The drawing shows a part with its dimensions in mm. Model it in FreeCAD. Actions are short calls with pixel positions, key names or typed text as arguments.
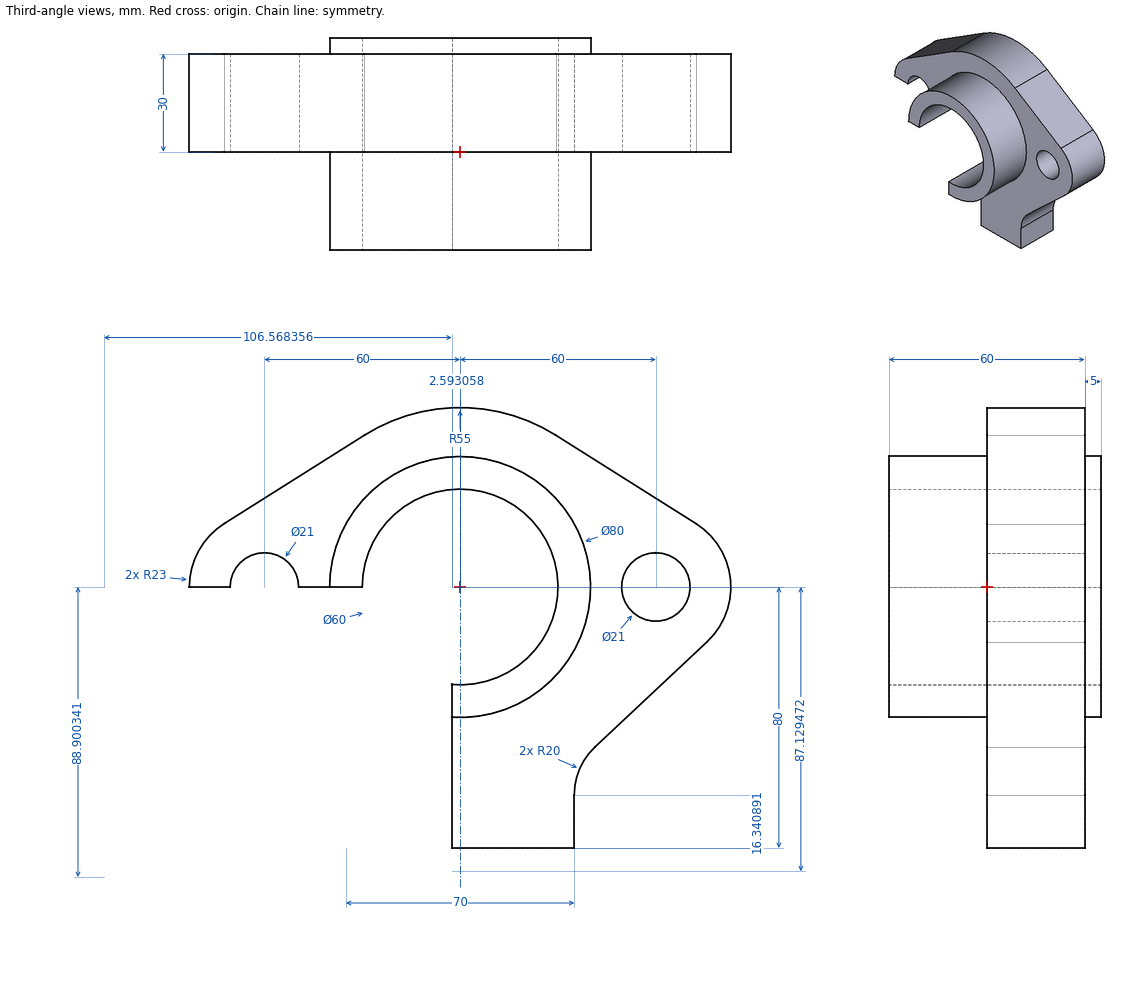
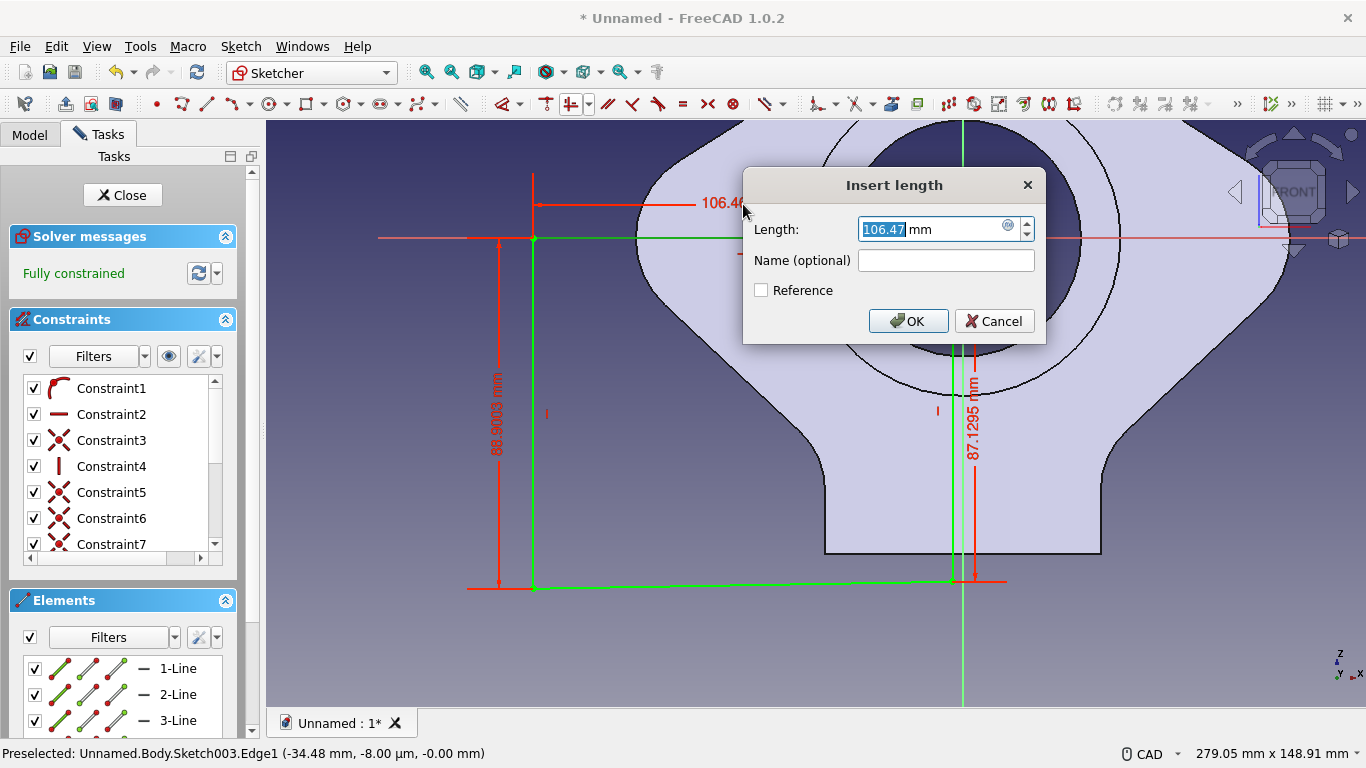
text(106.568356)
key(Return)
key(Escape)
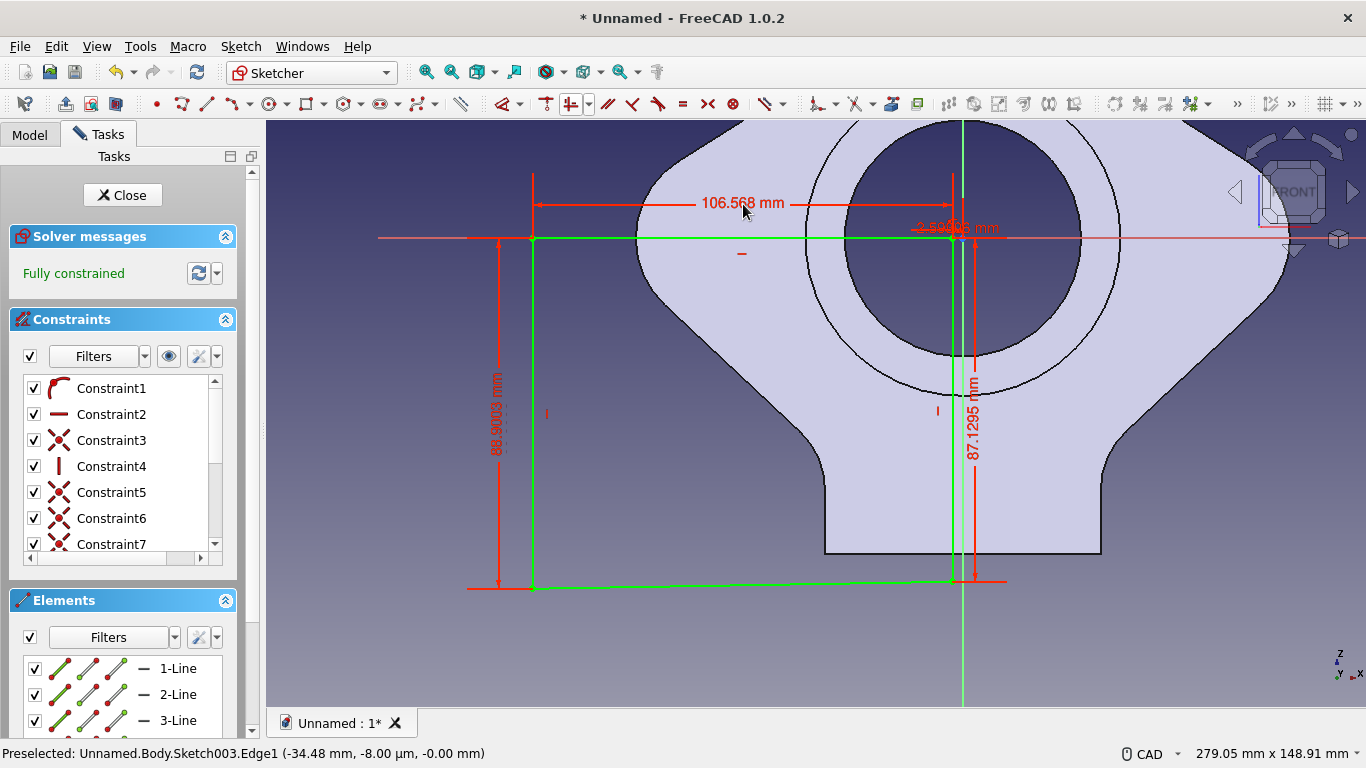
click(123, 195)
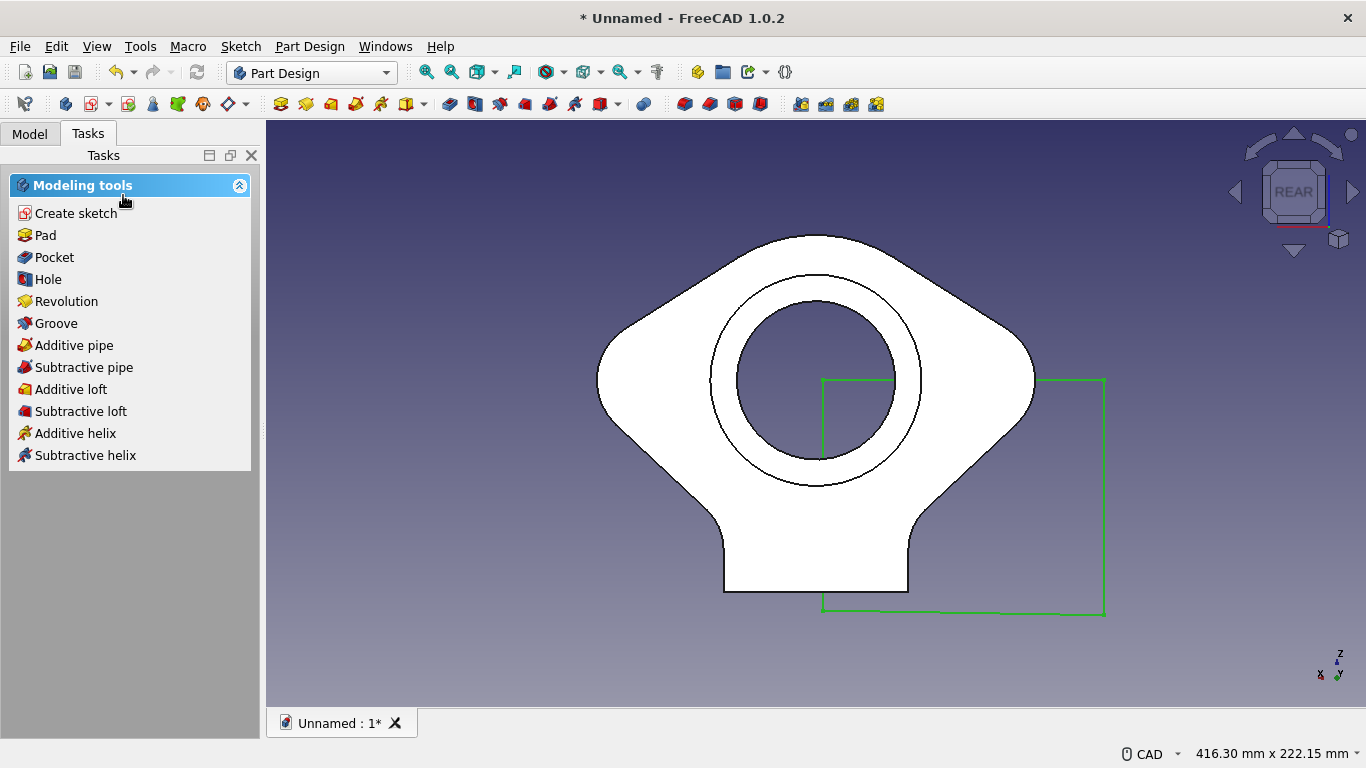
click(450, 104)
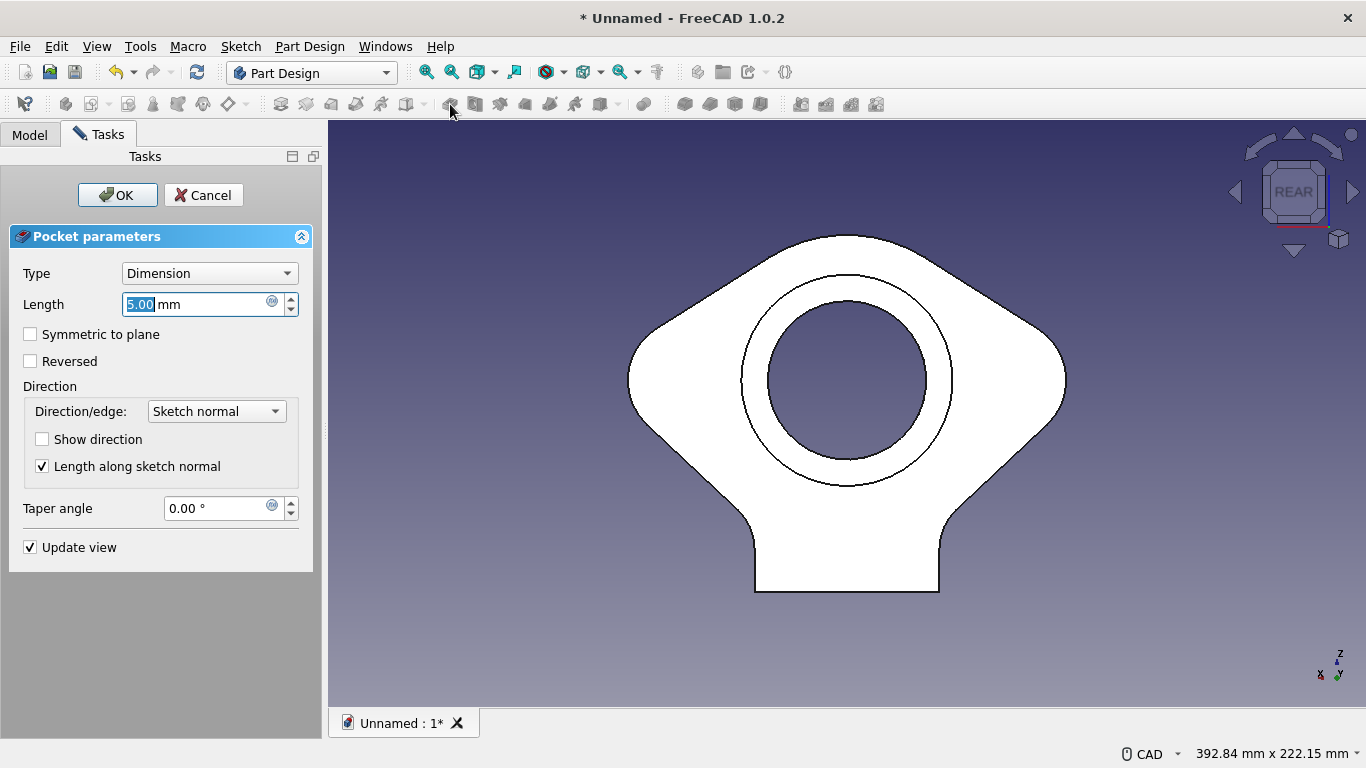
click(210, 274)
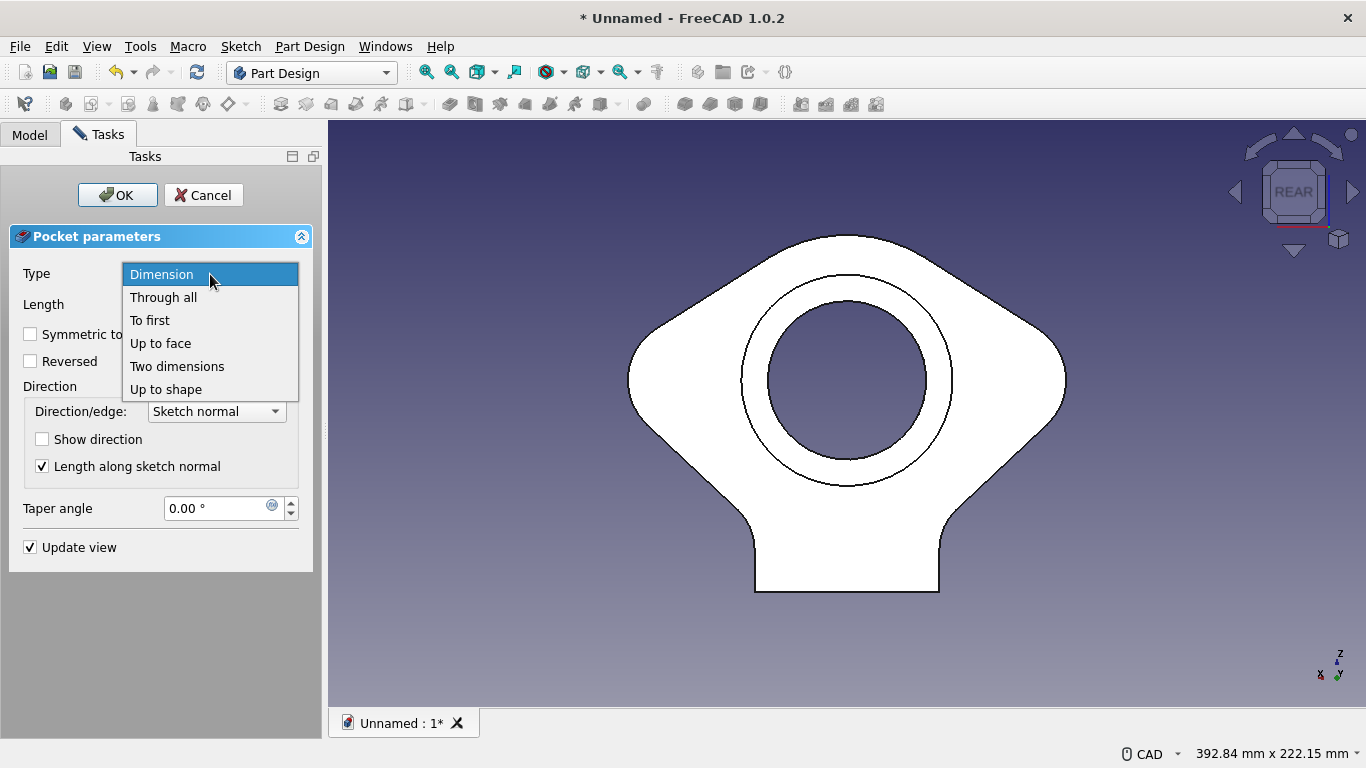
click(208, 366)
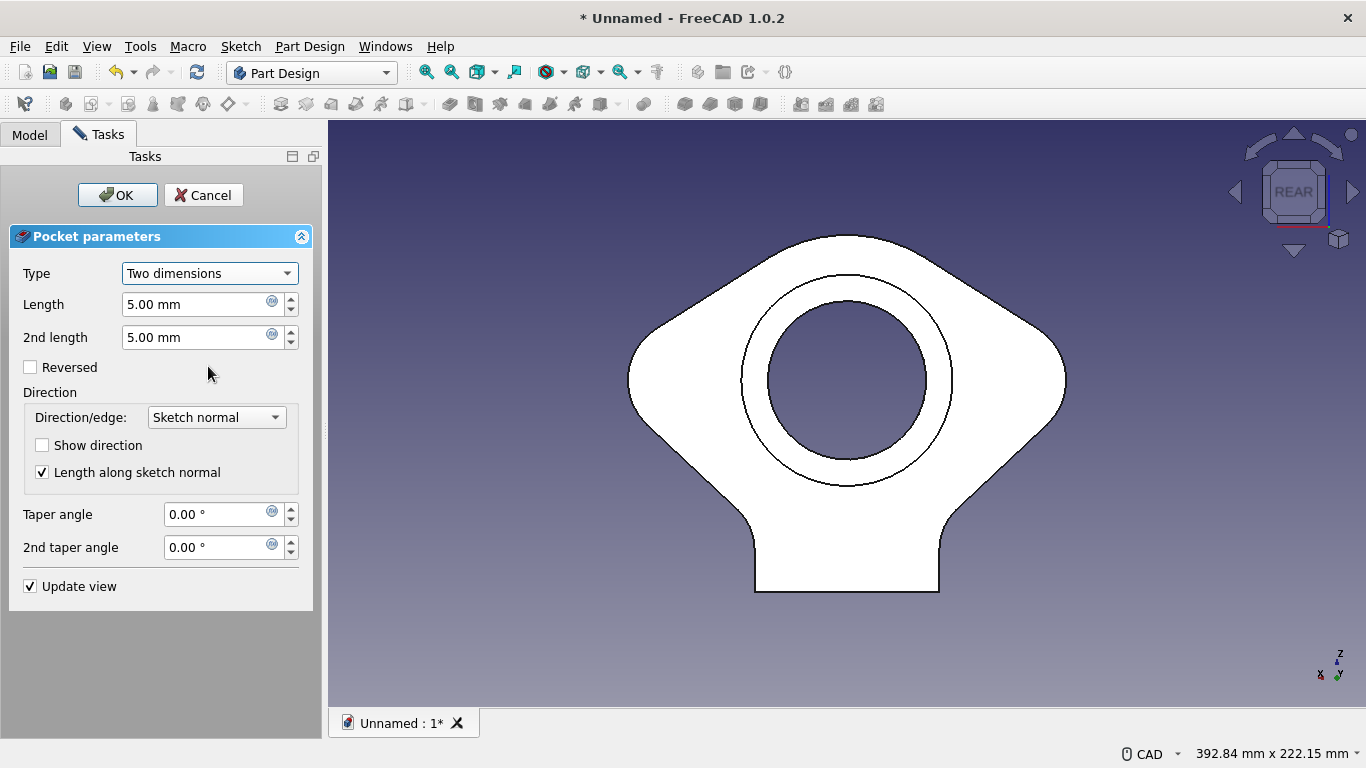
triple_click(204, 304)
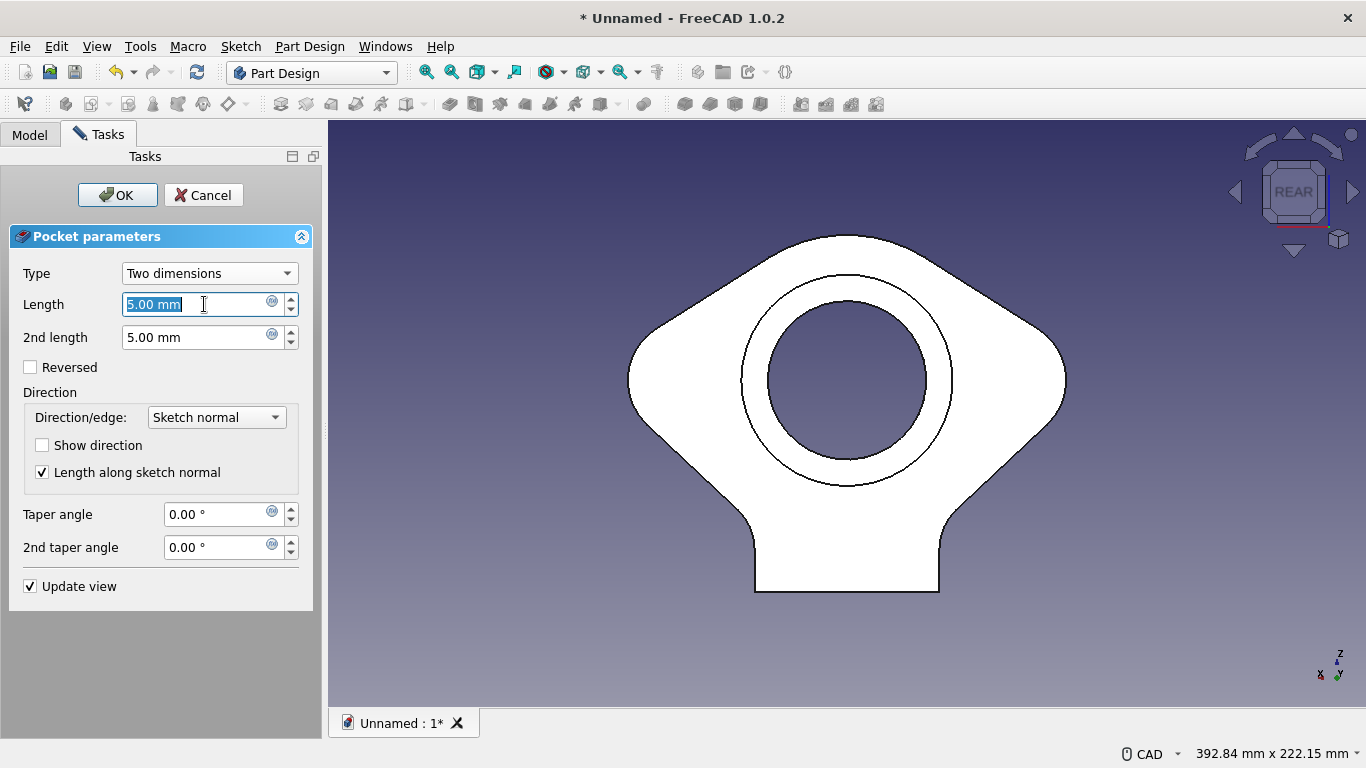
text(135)
key(Tab)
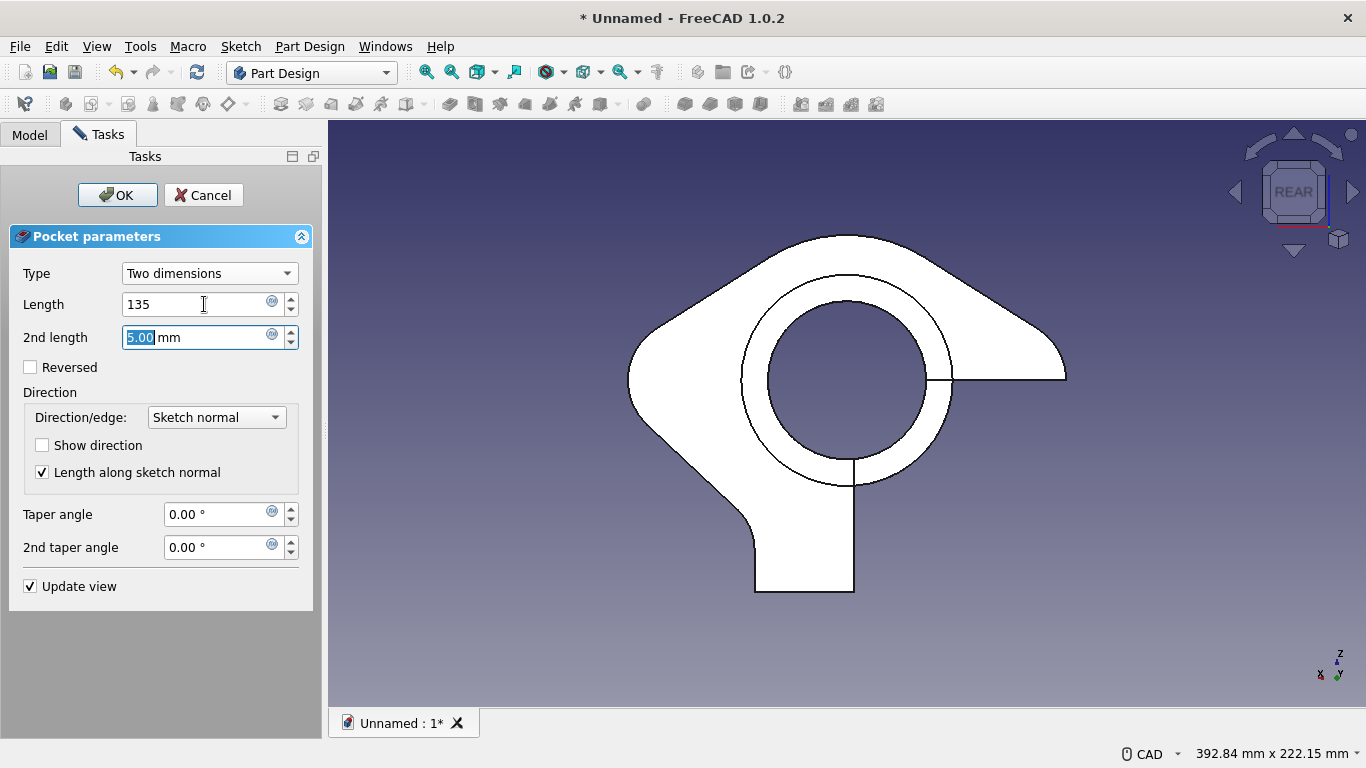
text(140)
key(Tab)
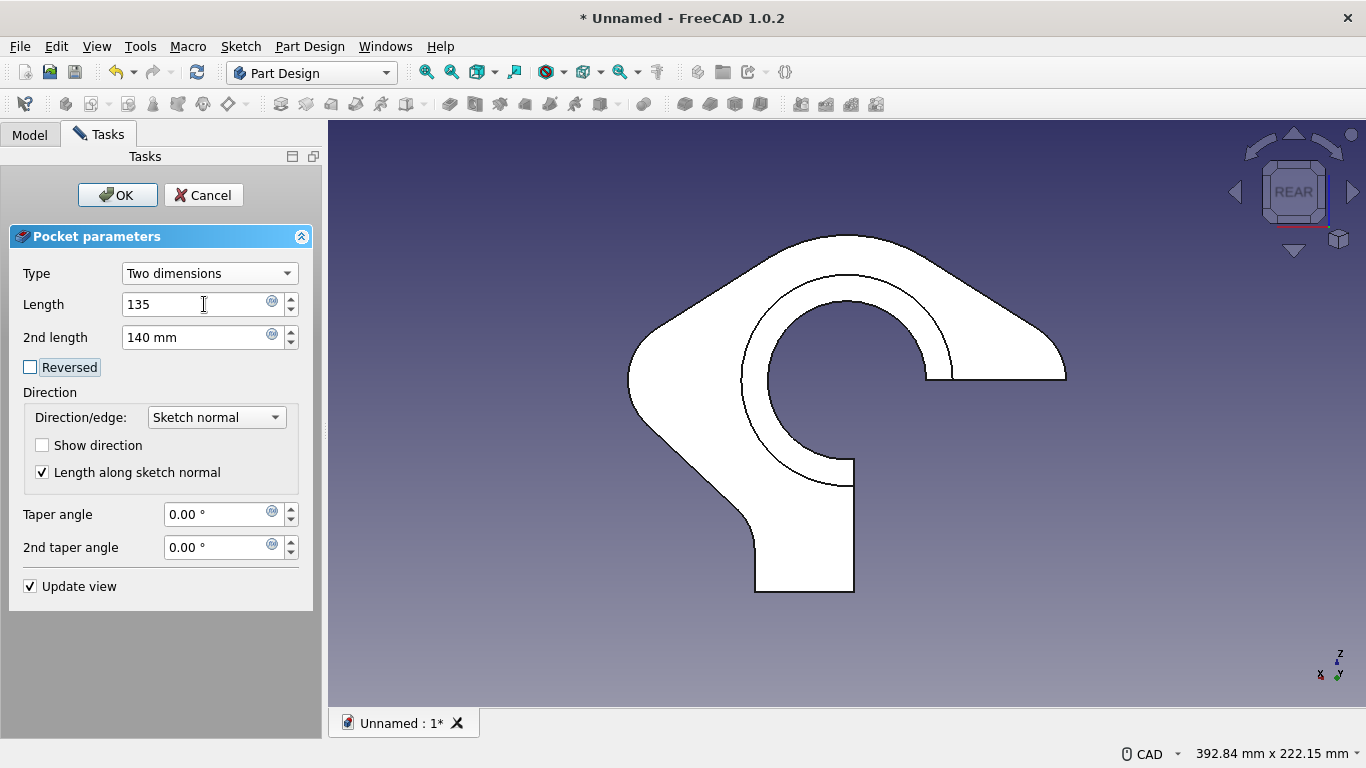
click(31, 367)